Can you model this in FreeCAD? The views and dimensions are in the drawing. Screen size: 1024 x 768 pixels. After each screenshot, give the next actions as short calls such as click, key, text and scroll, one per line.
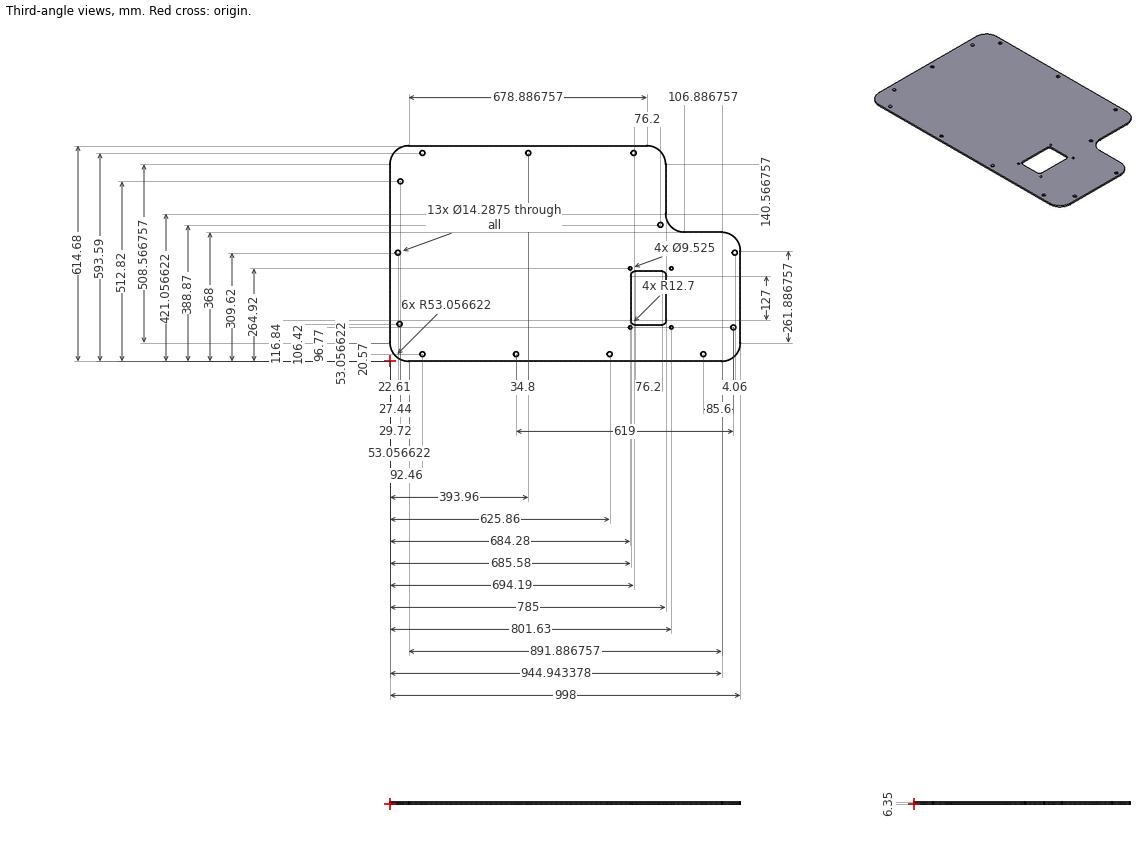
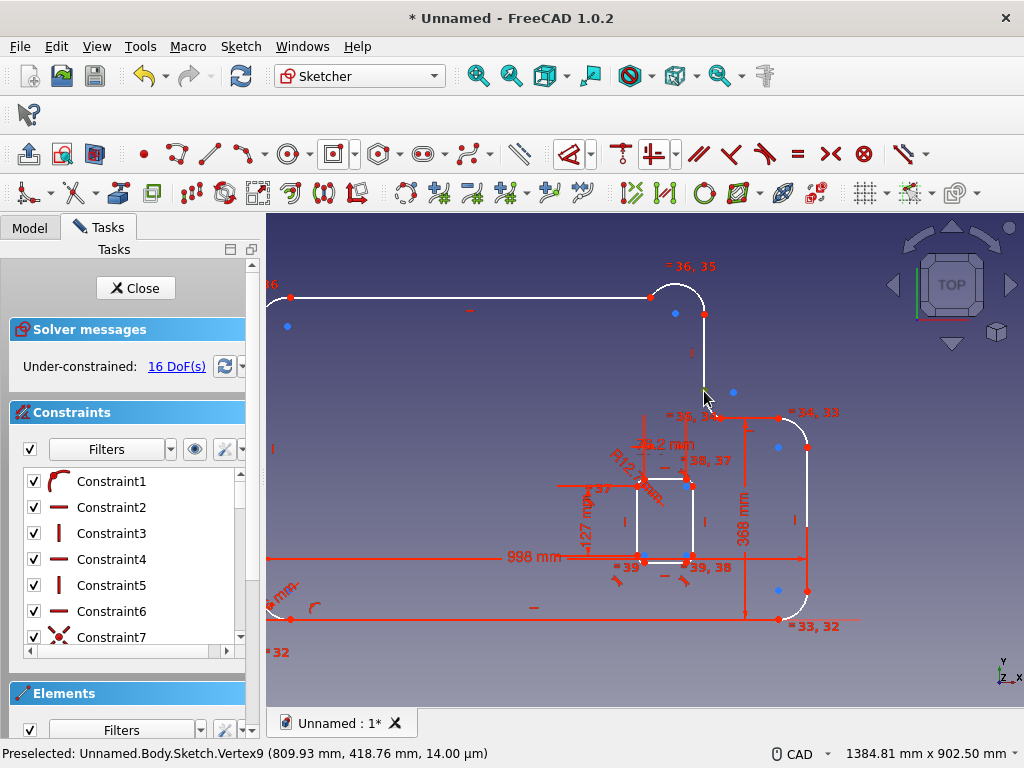
click(590, 154)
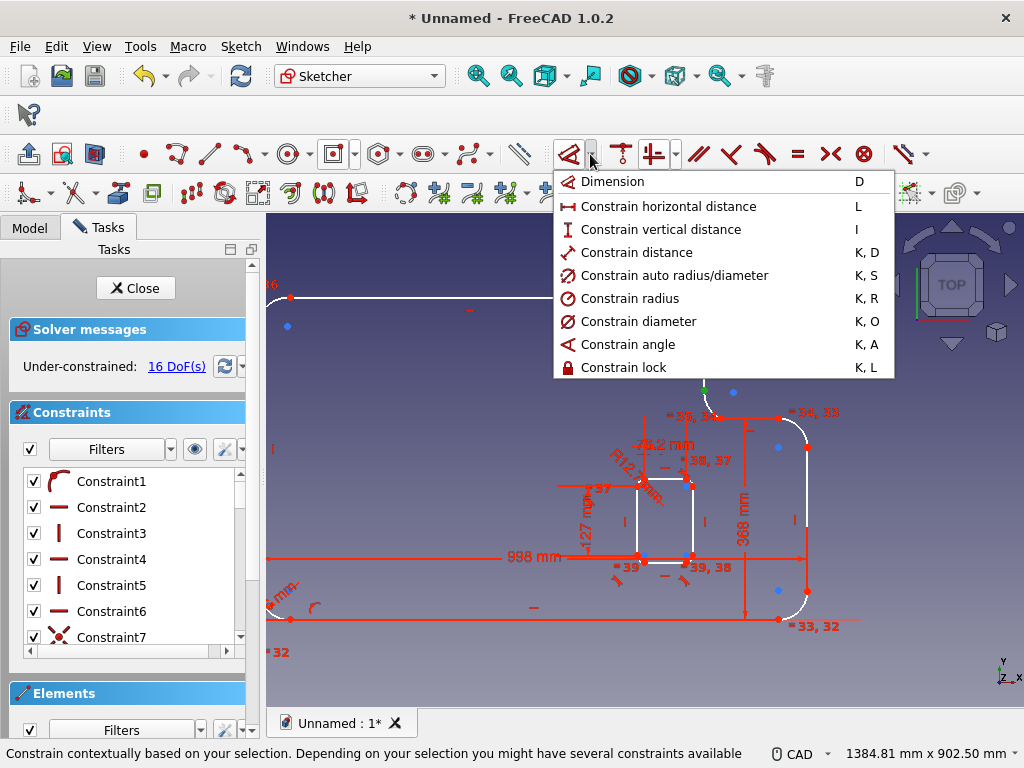
click(724, 206)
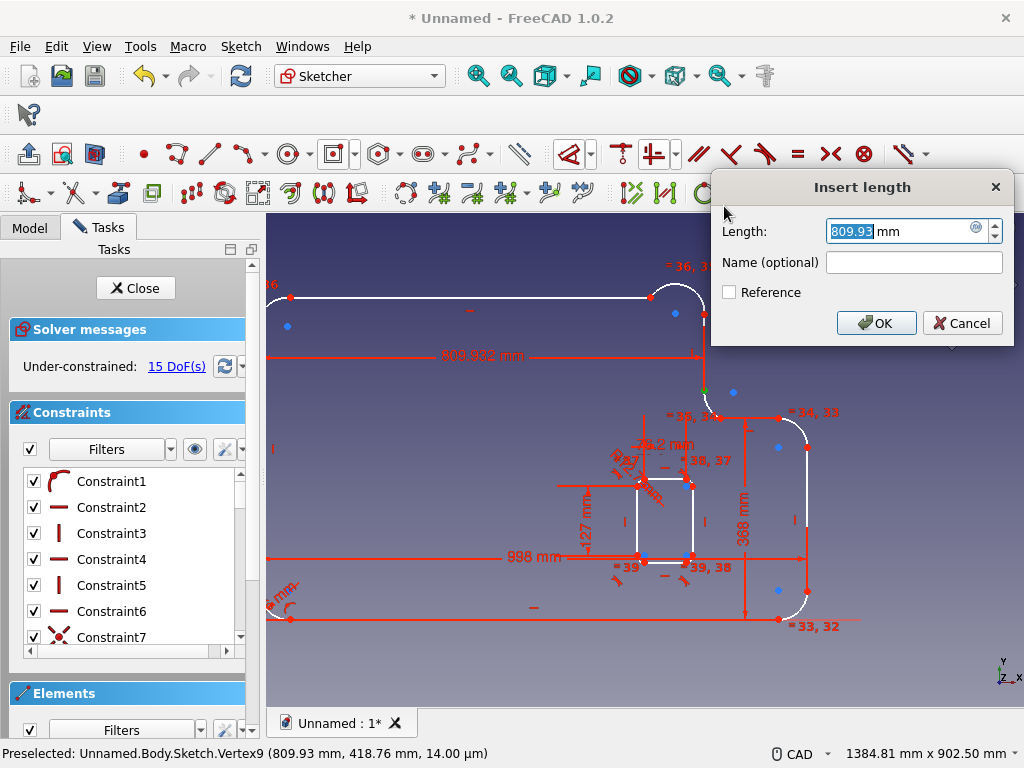
text(785)
key(Return)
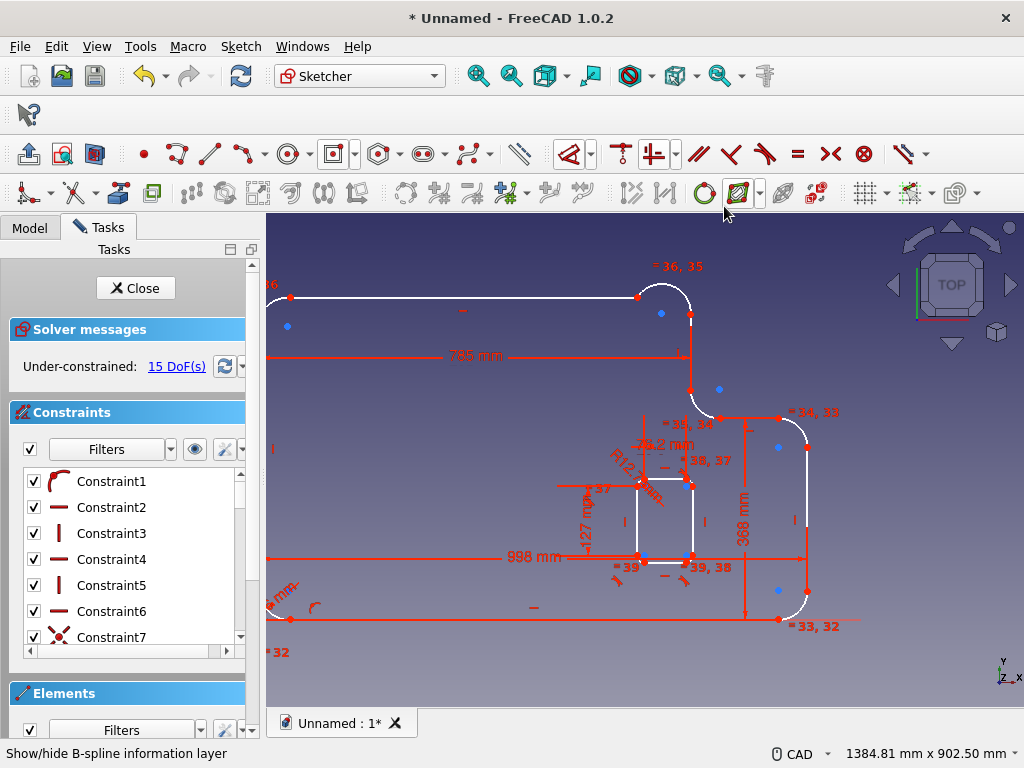
click(637, 298)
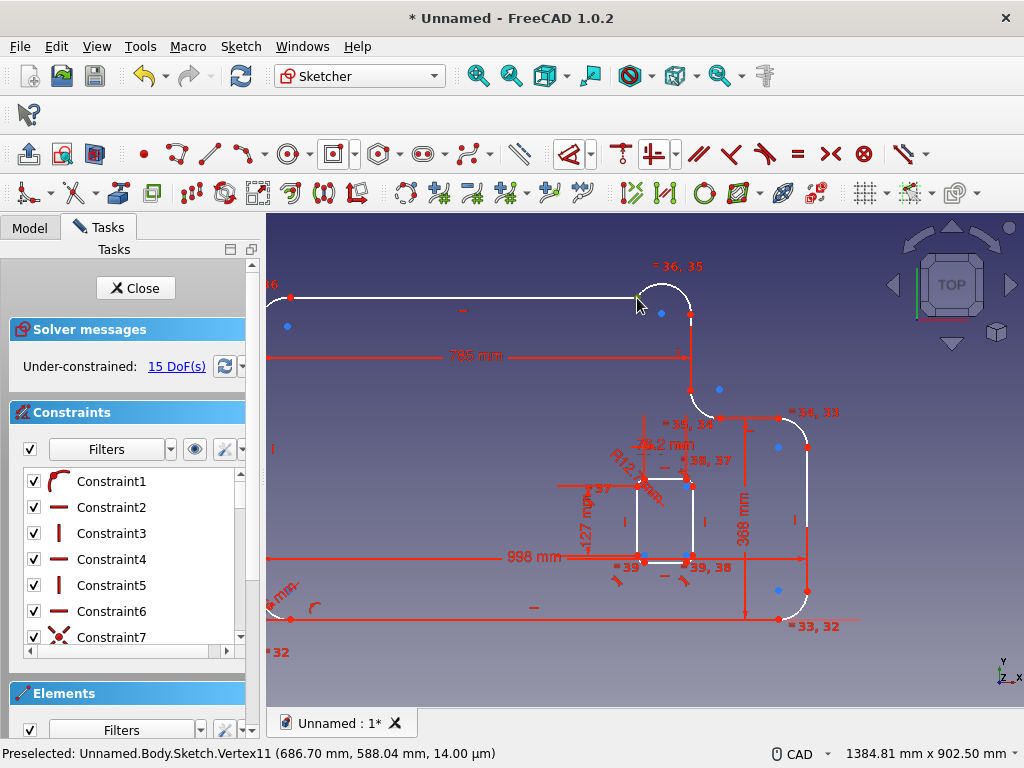
key(i)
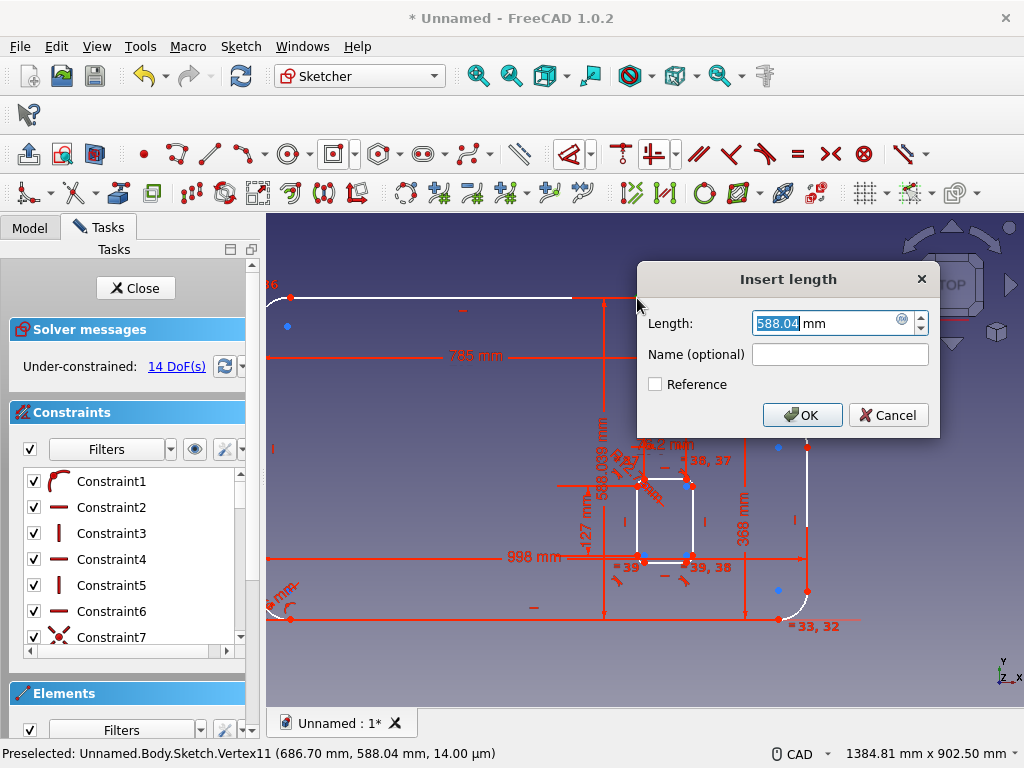
text(614.68)
key(Return)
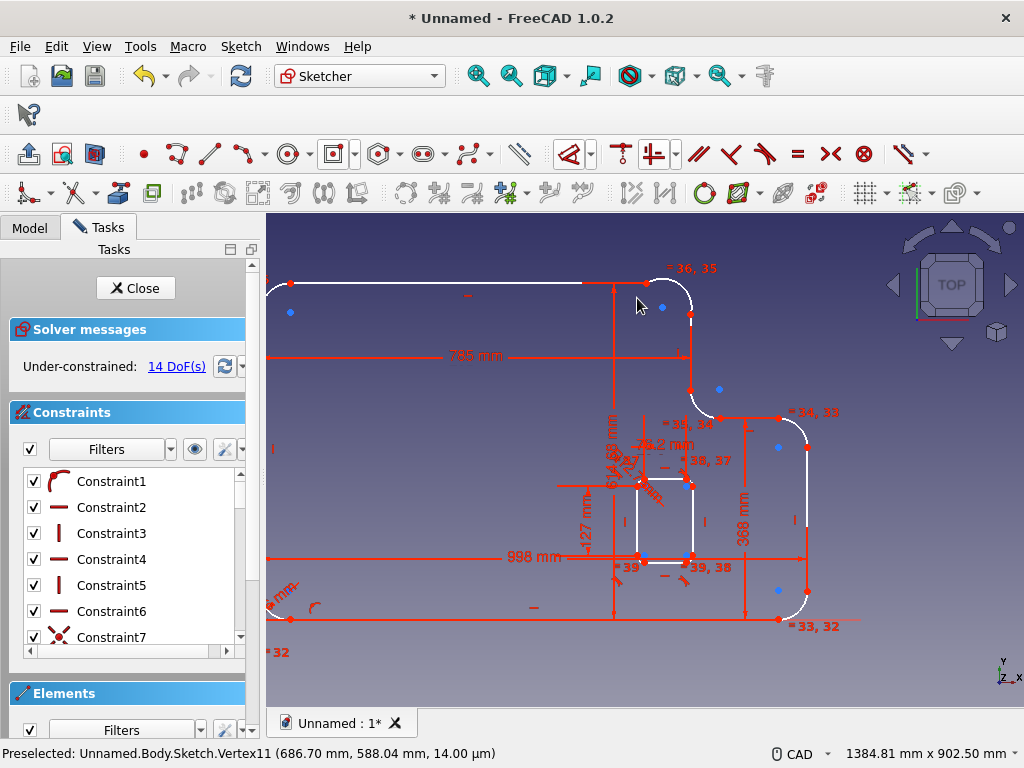
scroll(637, 556, up, 3)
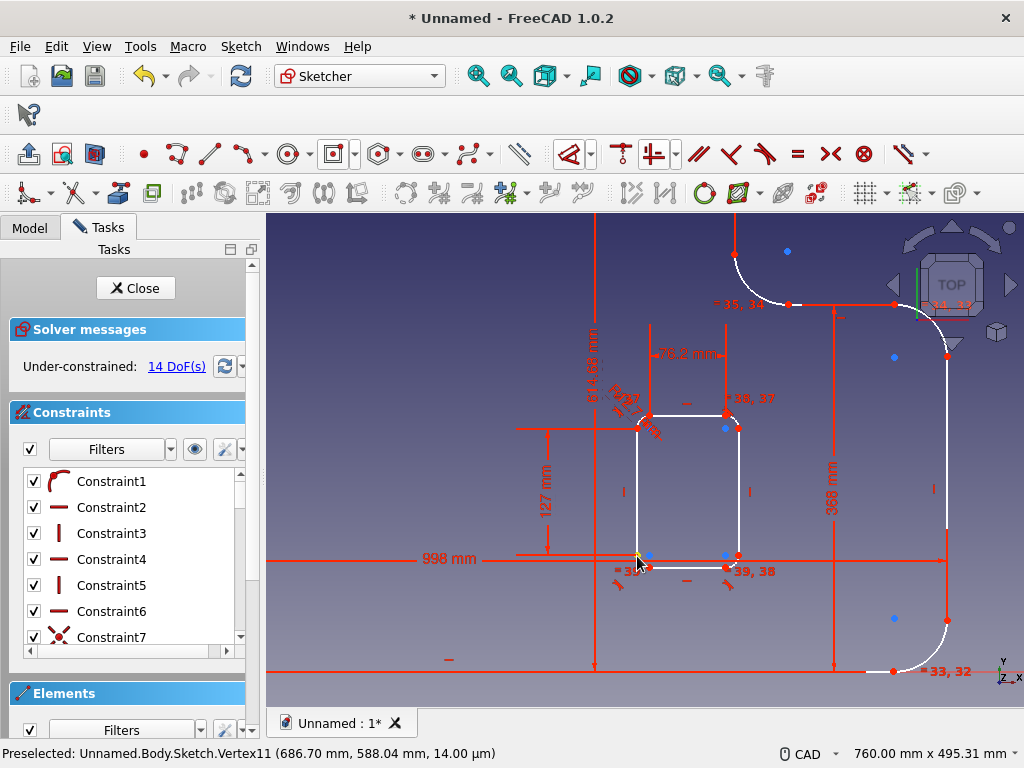
click(637, 555)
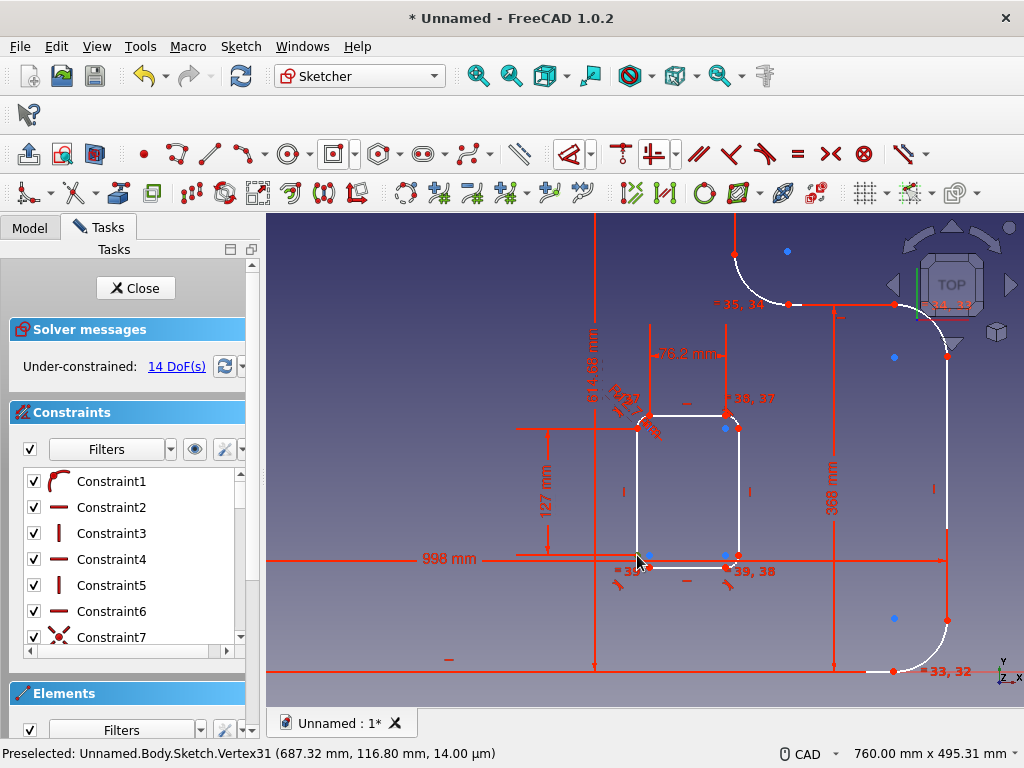
click(590, 154)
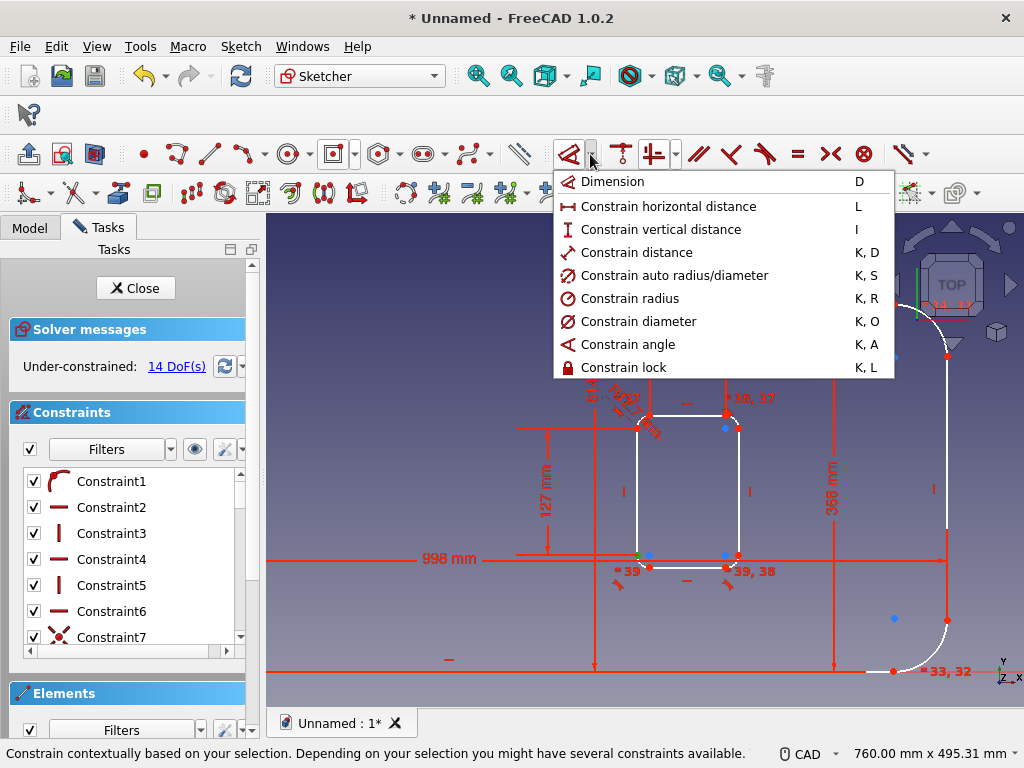
click(724, 206)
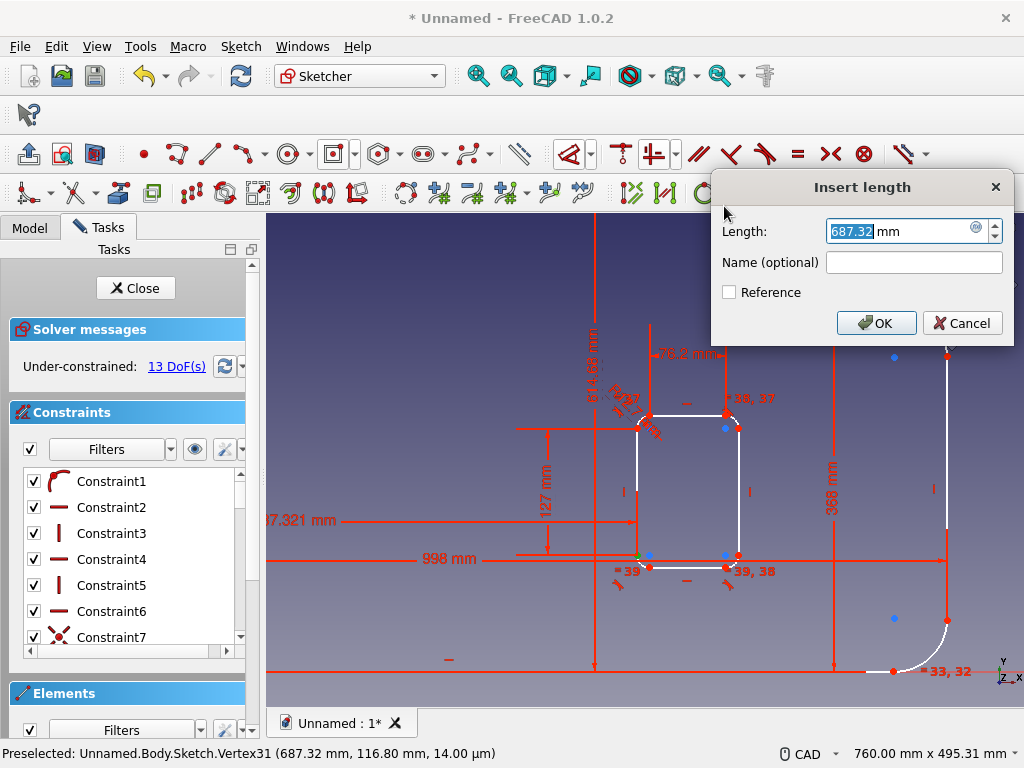
text(685.58)
key(Return)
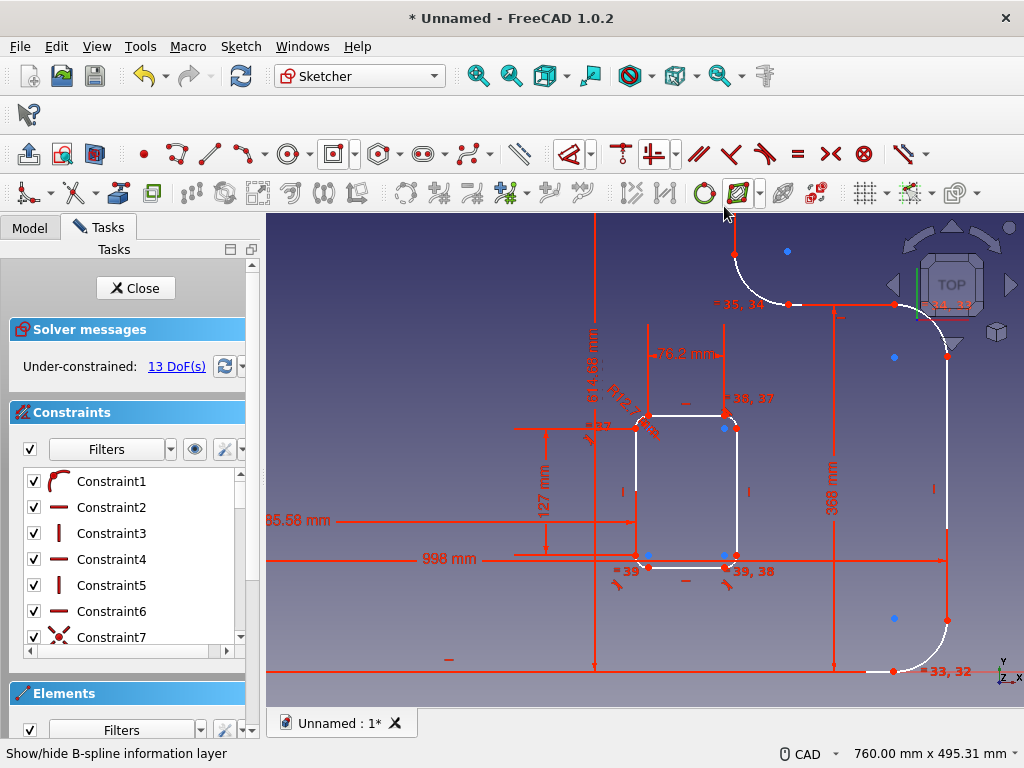
click(636, 555)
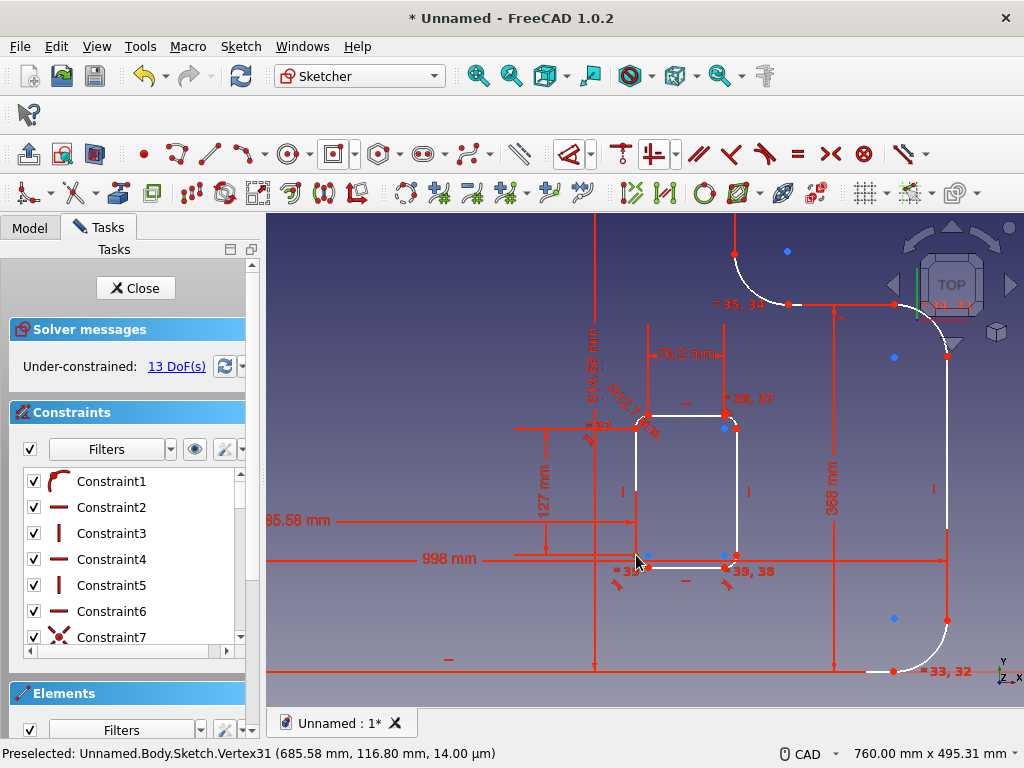
click(590, 154)